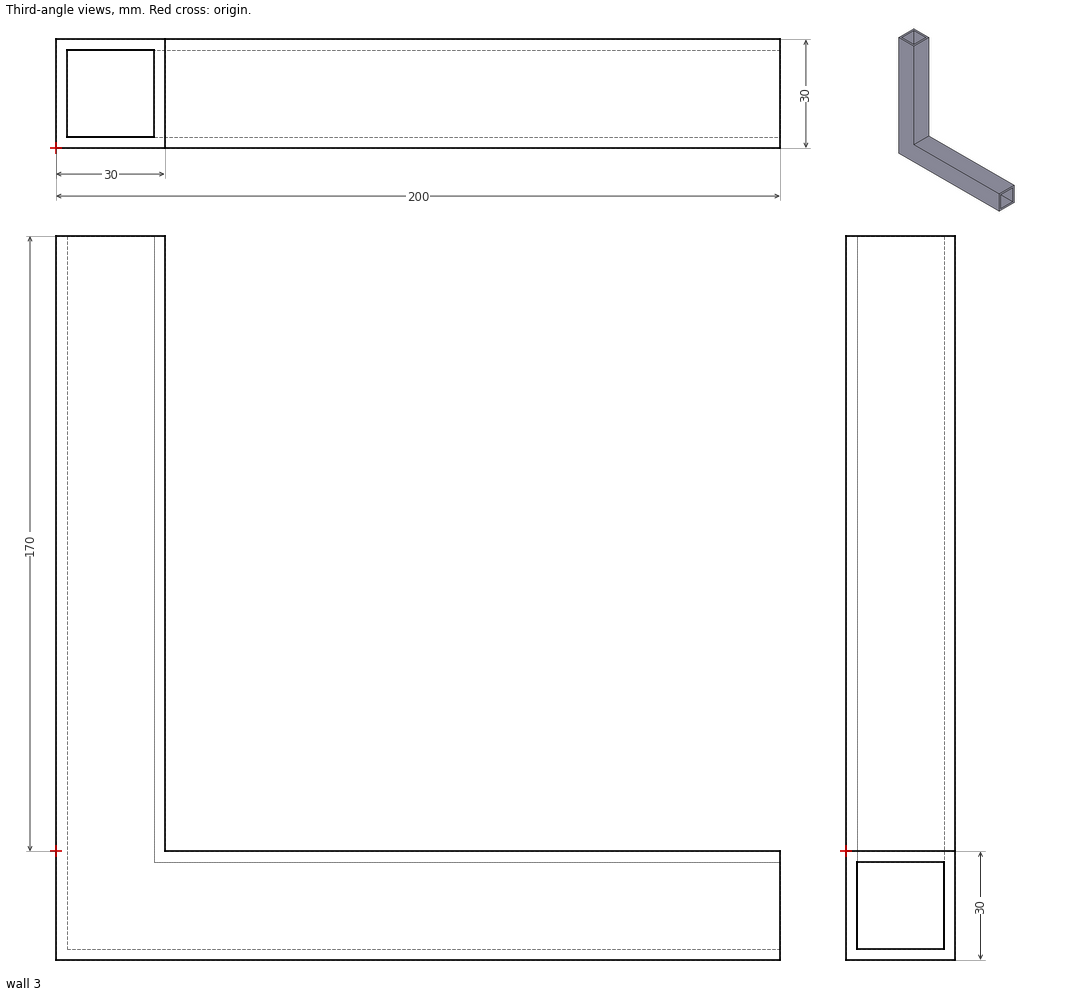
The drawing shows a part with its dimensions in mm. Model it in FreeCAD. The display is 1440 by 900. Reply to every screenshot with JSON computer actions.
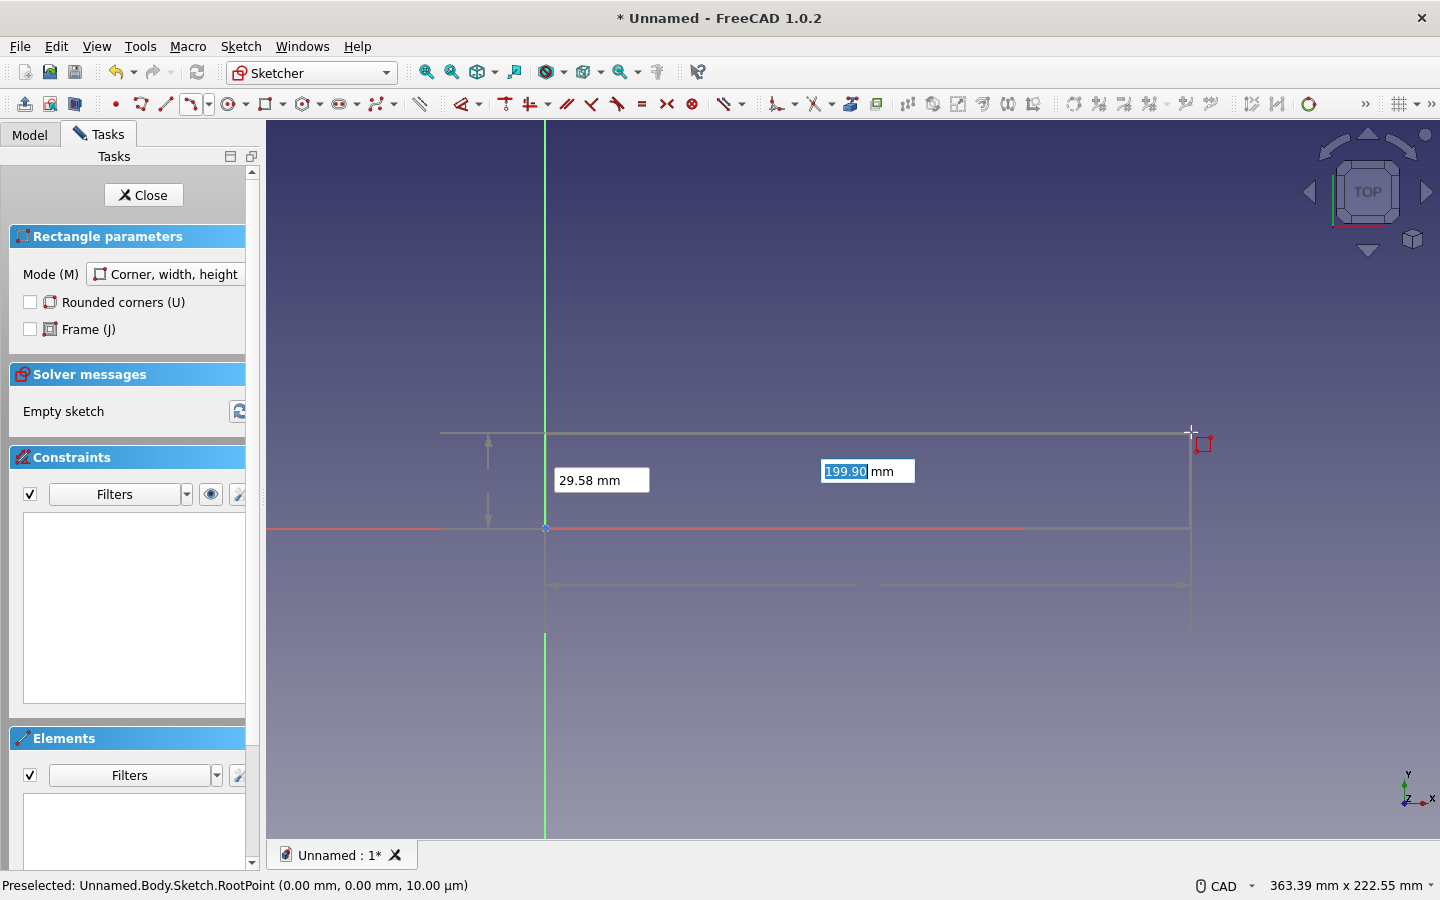
{"action": "type", "text": "200"}
{"action": "key", "text": "Tab"}
{"action": "type", "text": "30"}
{"action": "key", "text": "Return"}
{"action": "key", "text": "Escape"}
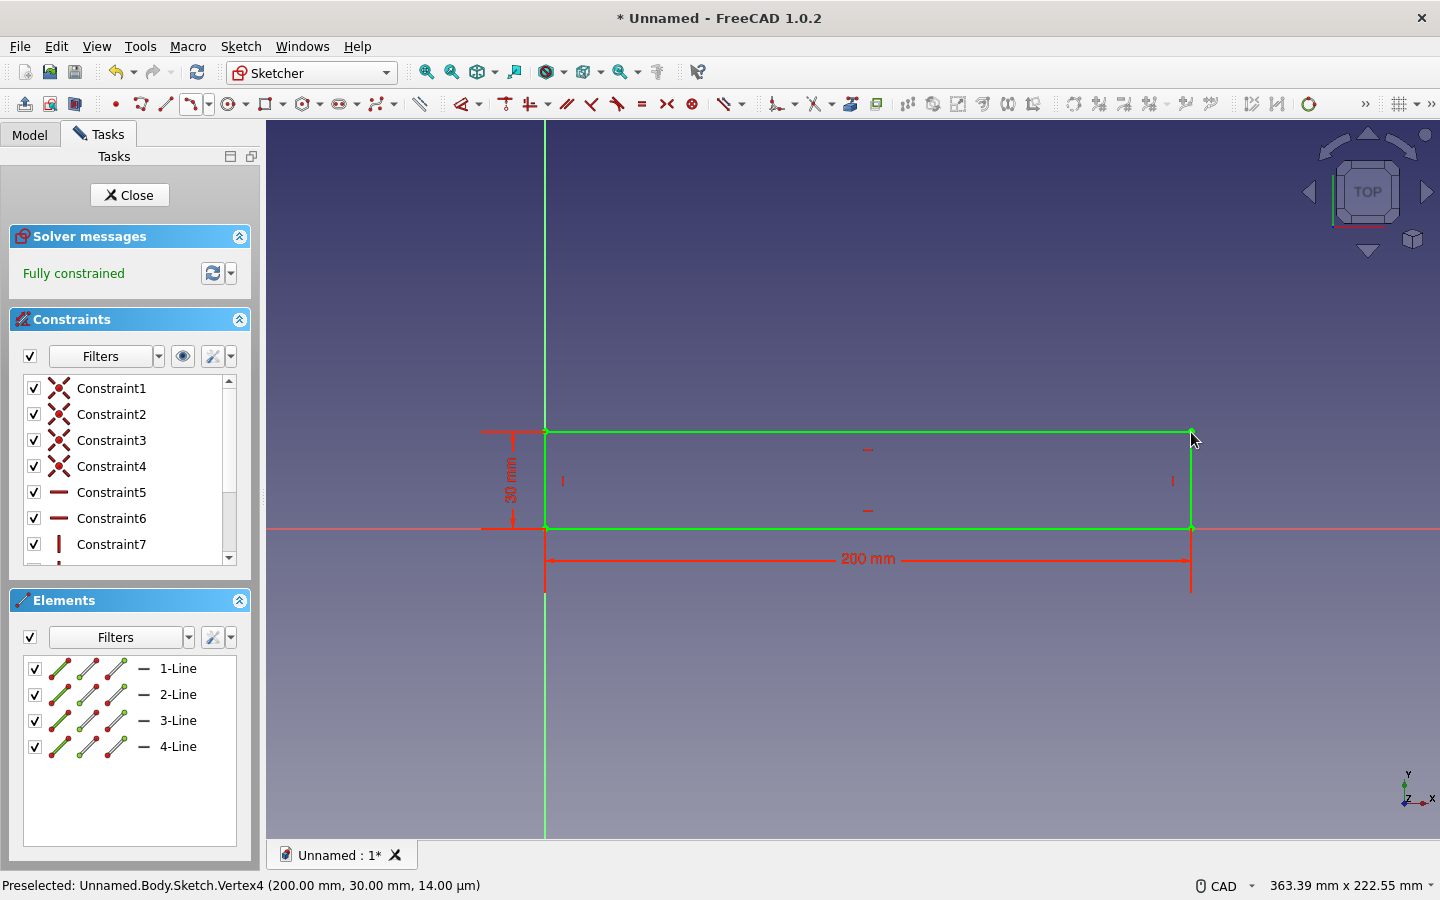
{"action": "left_click", "coordinate": [130, 195]}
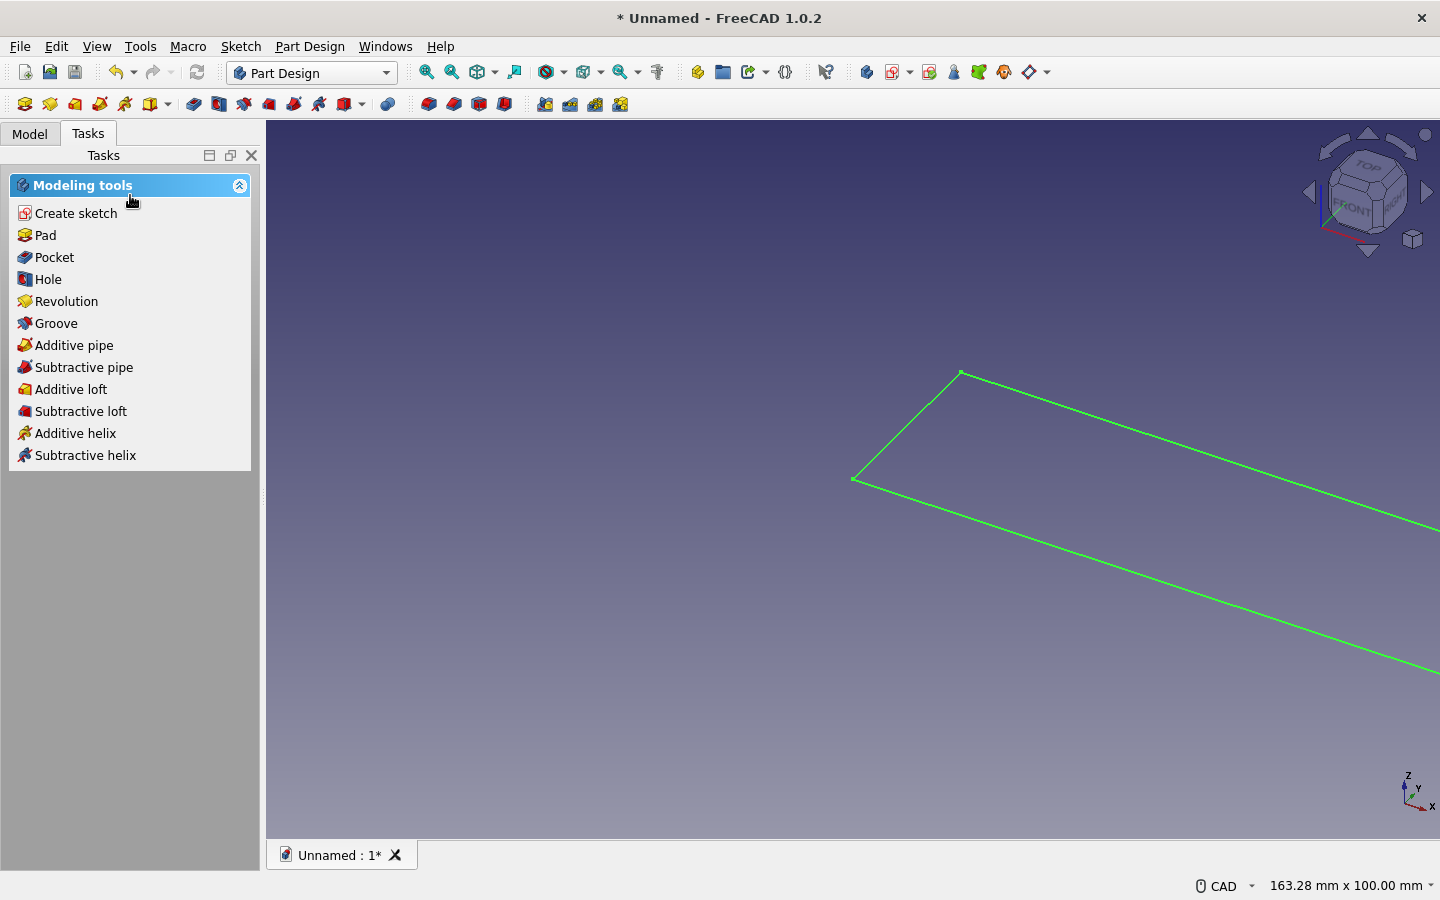
{"action": "left_click", "coordinate": [25, 104]}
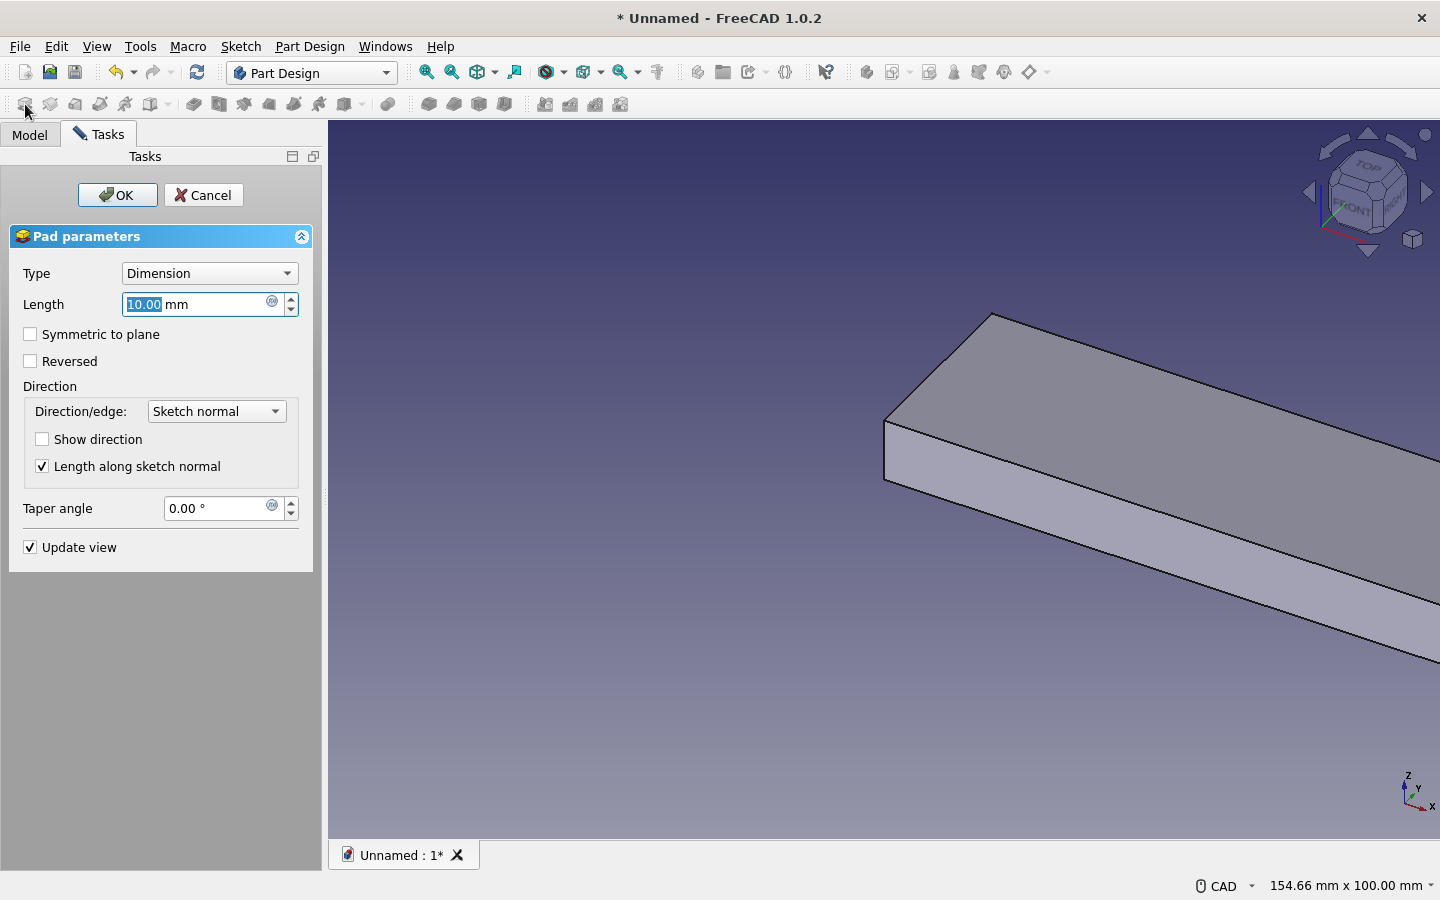
{"action": "type", "text": "30"}
{"action": "key", "text": "Tab"}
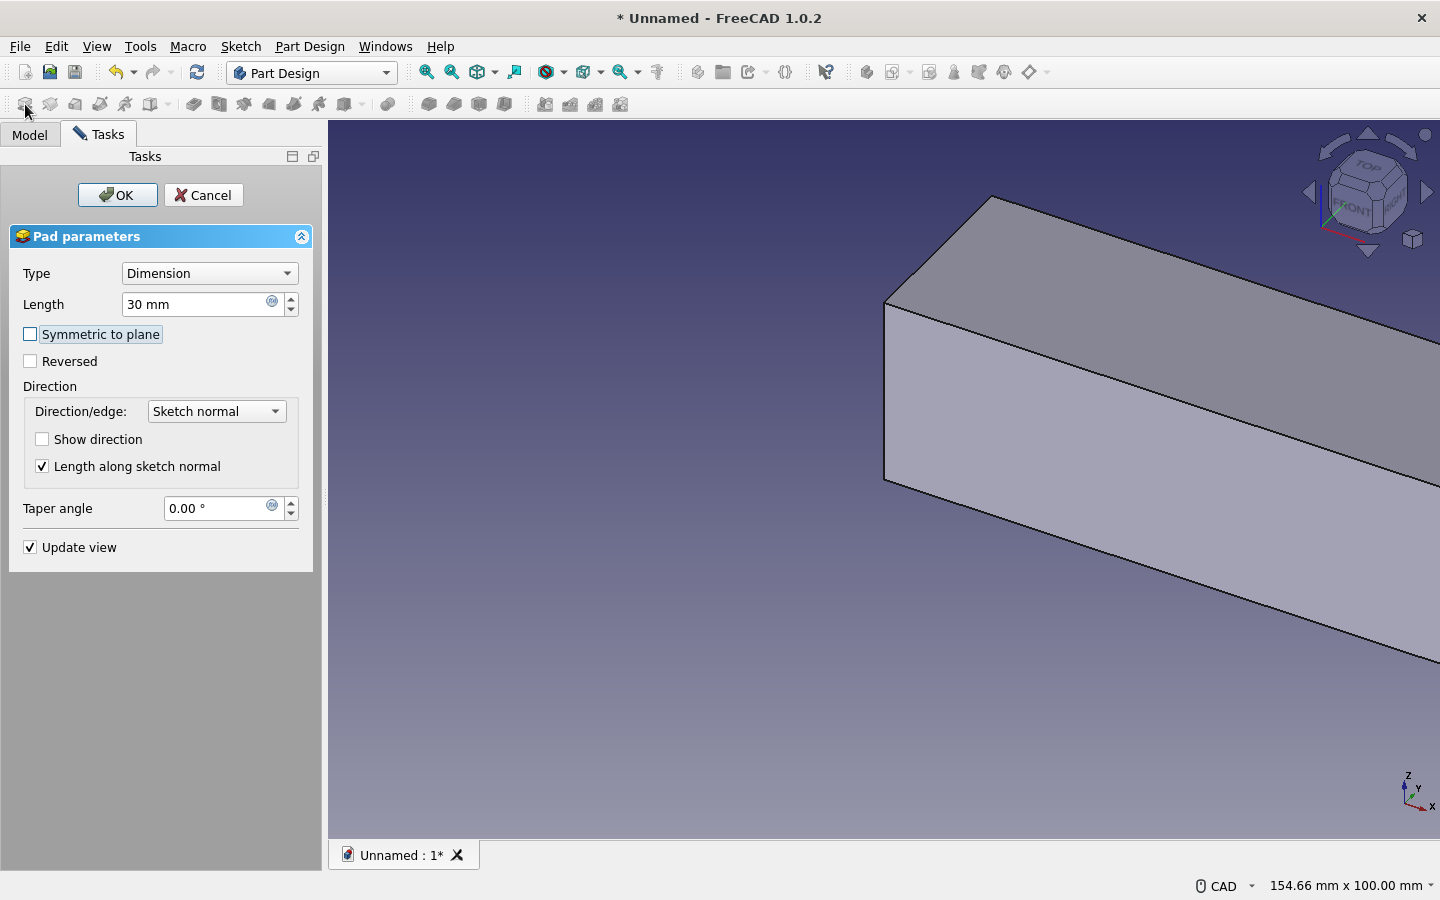
{"action": "left_click", "coordinate": [31, 361]}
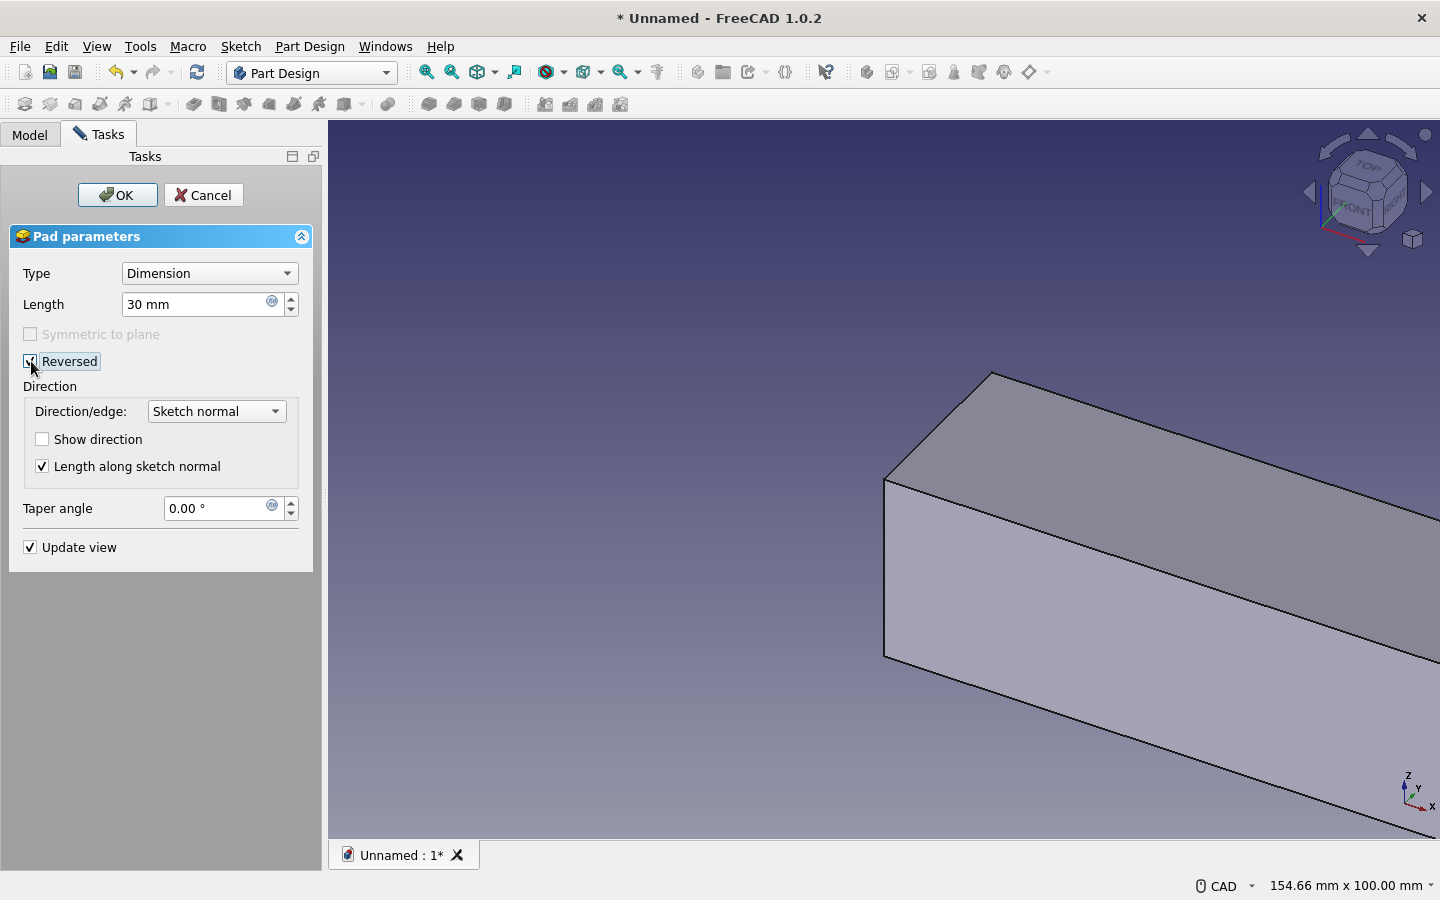
{"action": "left_click", "coordinate": [118, 195]}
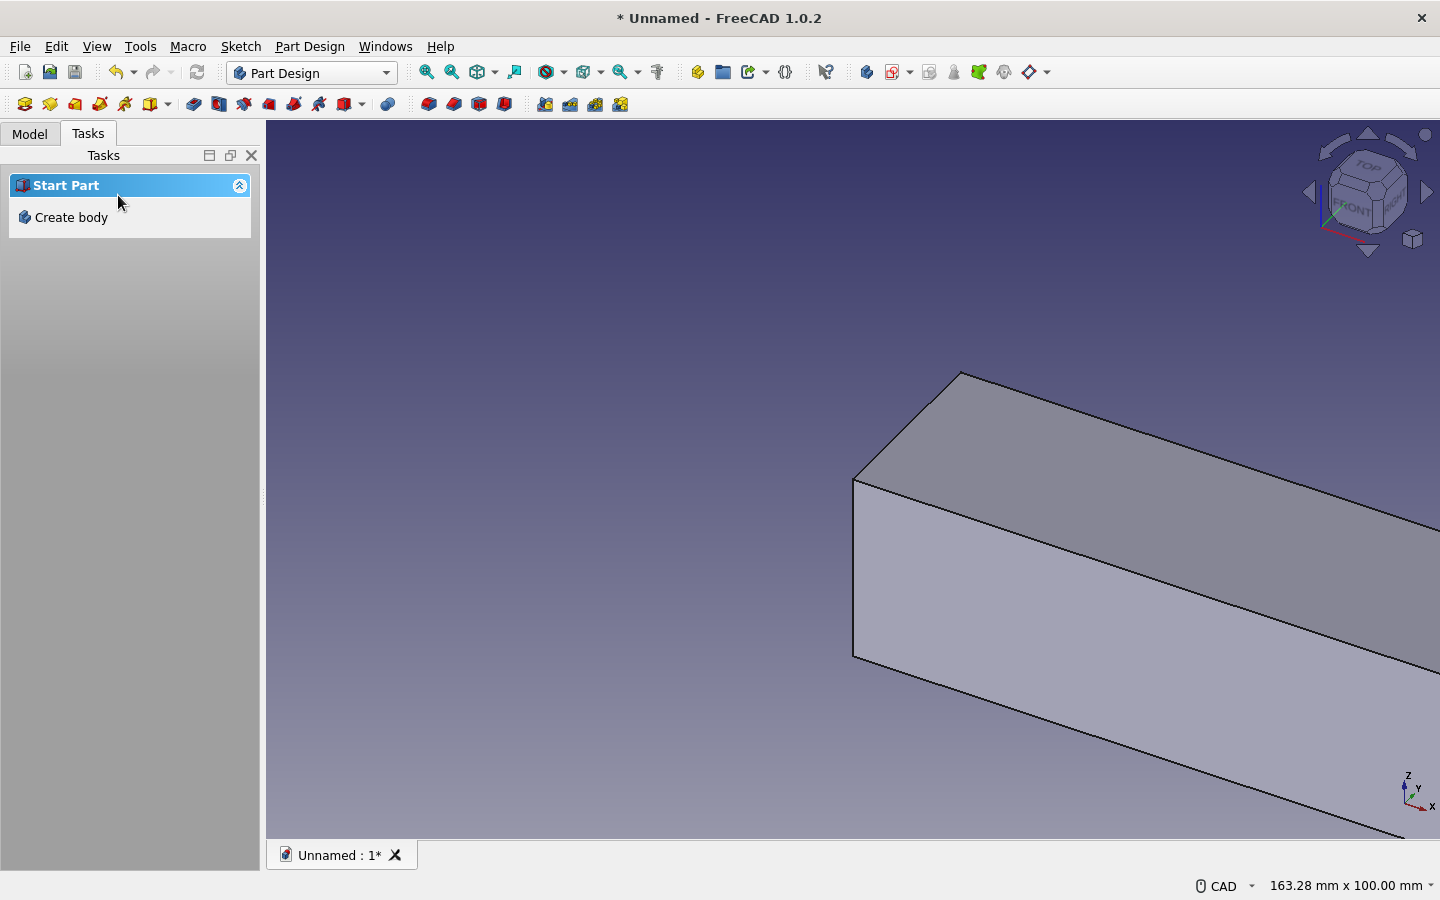
{"action": "left_click", "coordinate": [427, 72]}